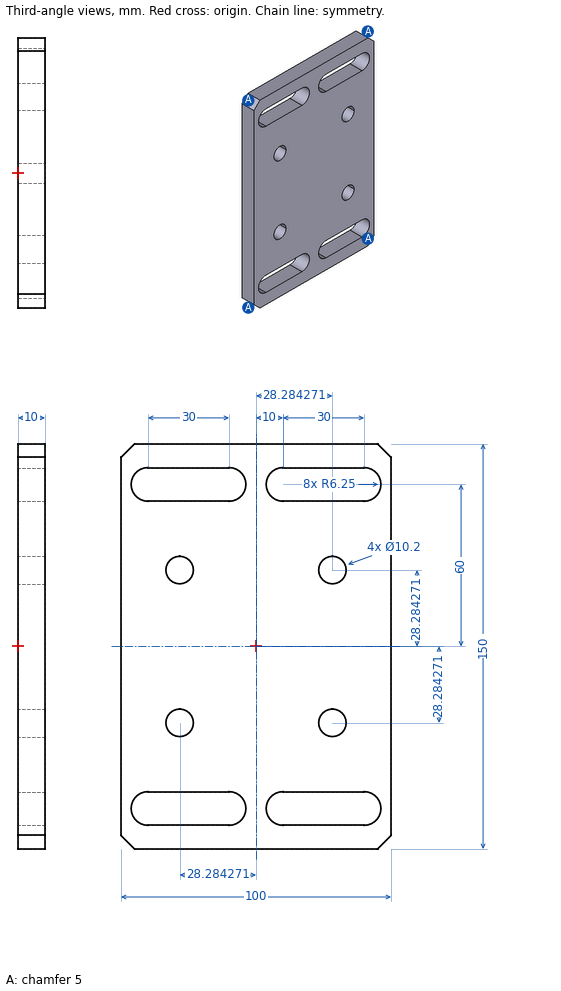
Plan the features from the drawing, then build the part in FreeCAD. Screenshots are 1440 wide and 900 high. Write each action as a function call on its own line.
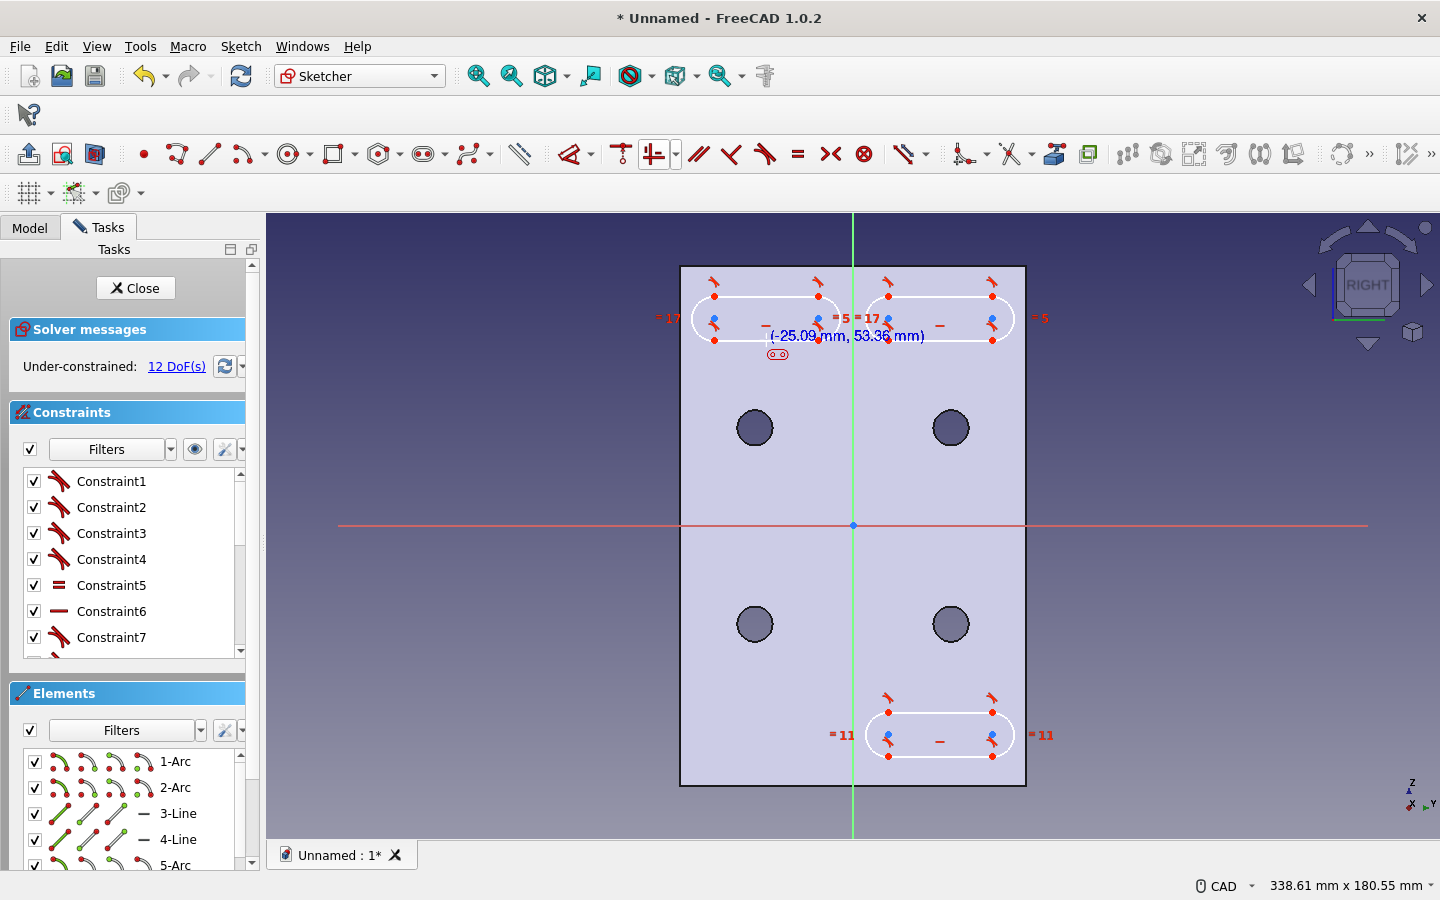
click(714, 734)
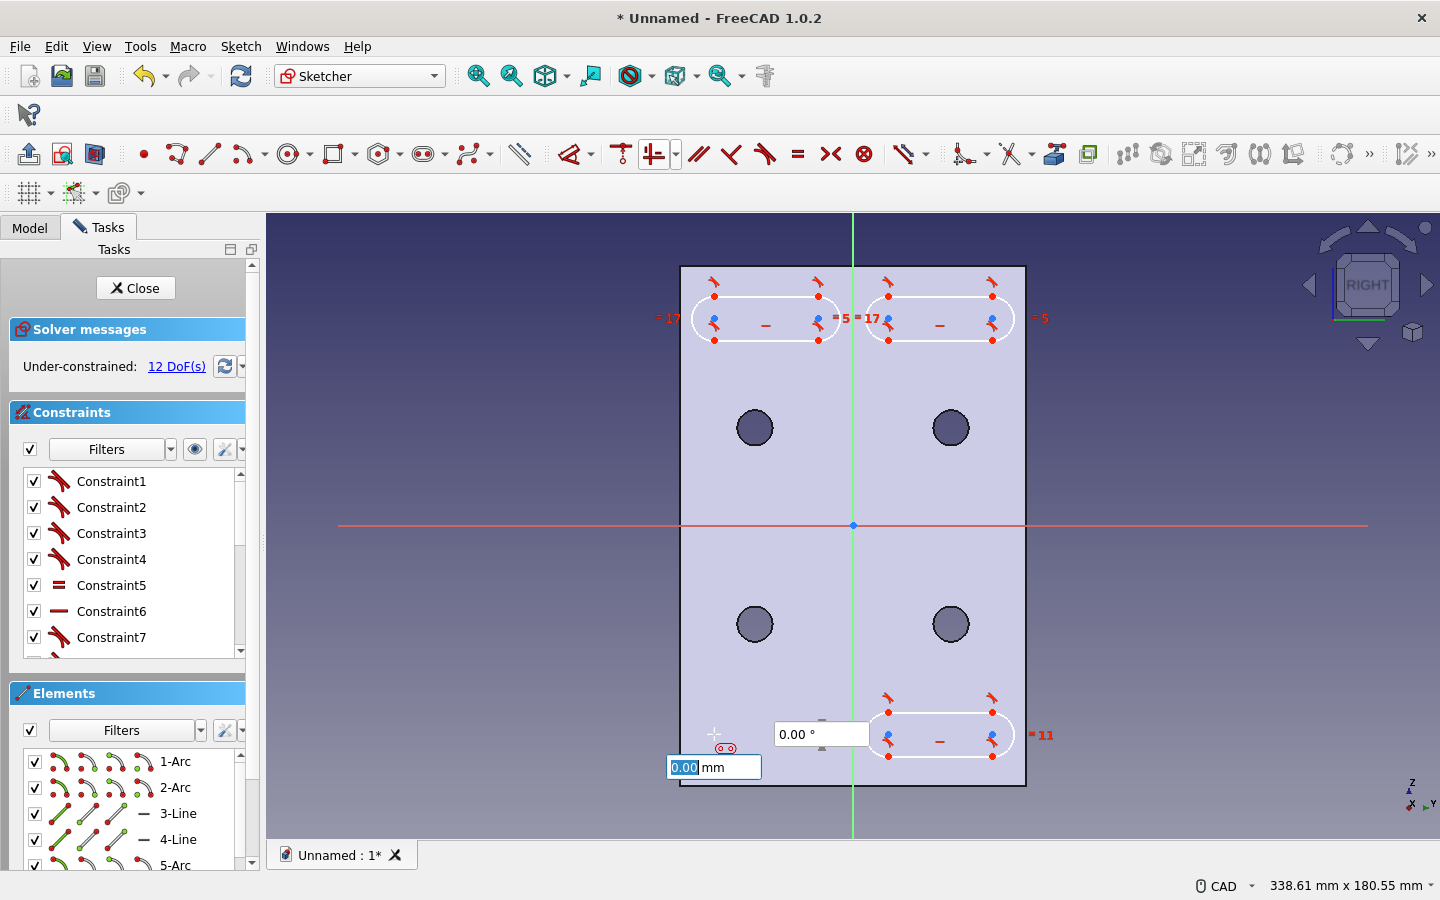
click(818, 734)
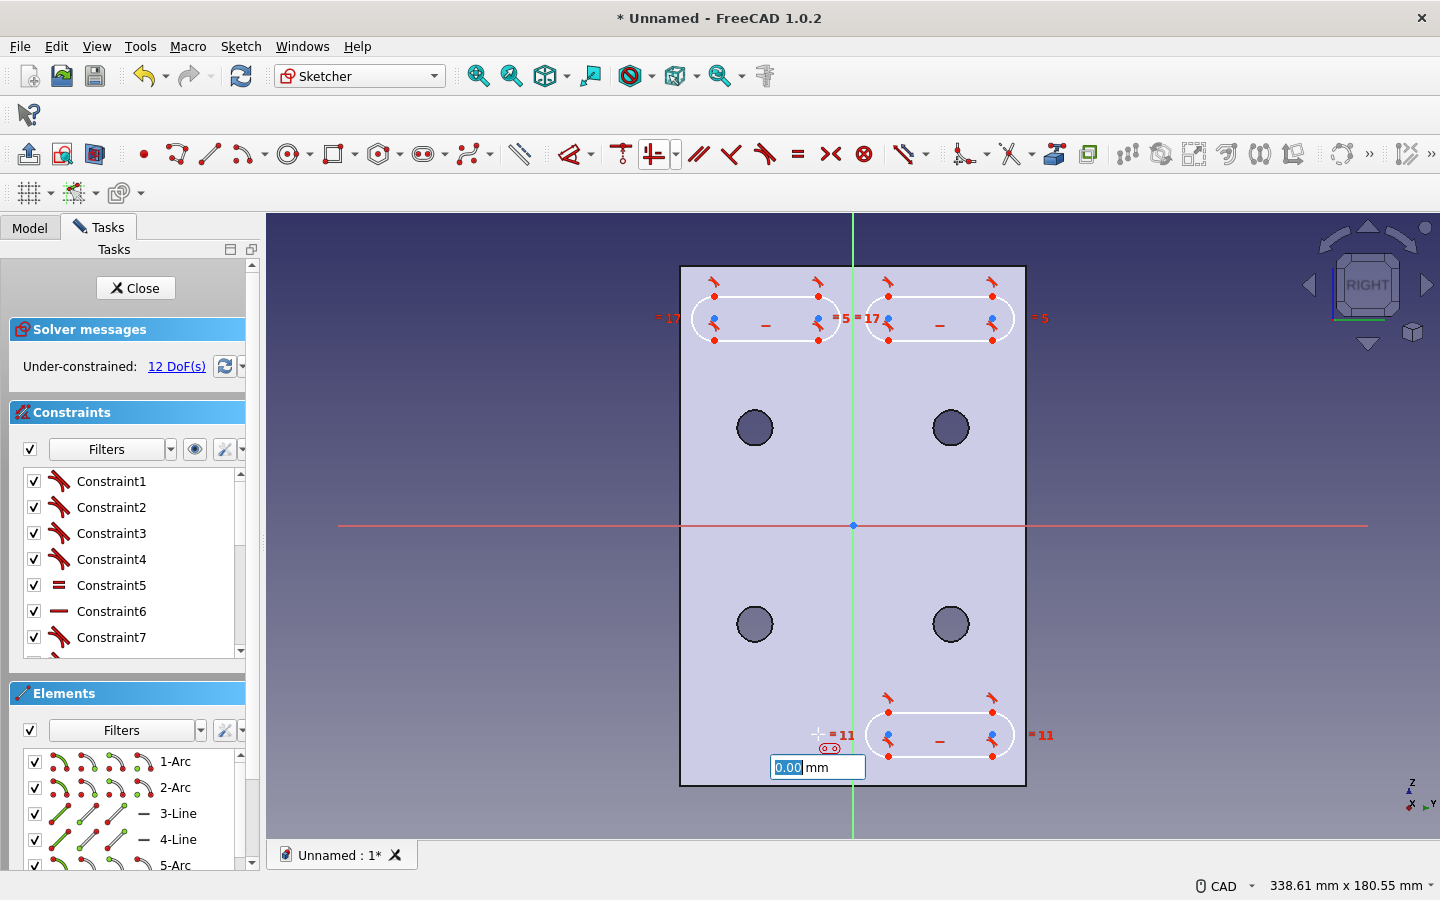
click(766, 712)
key(Escape)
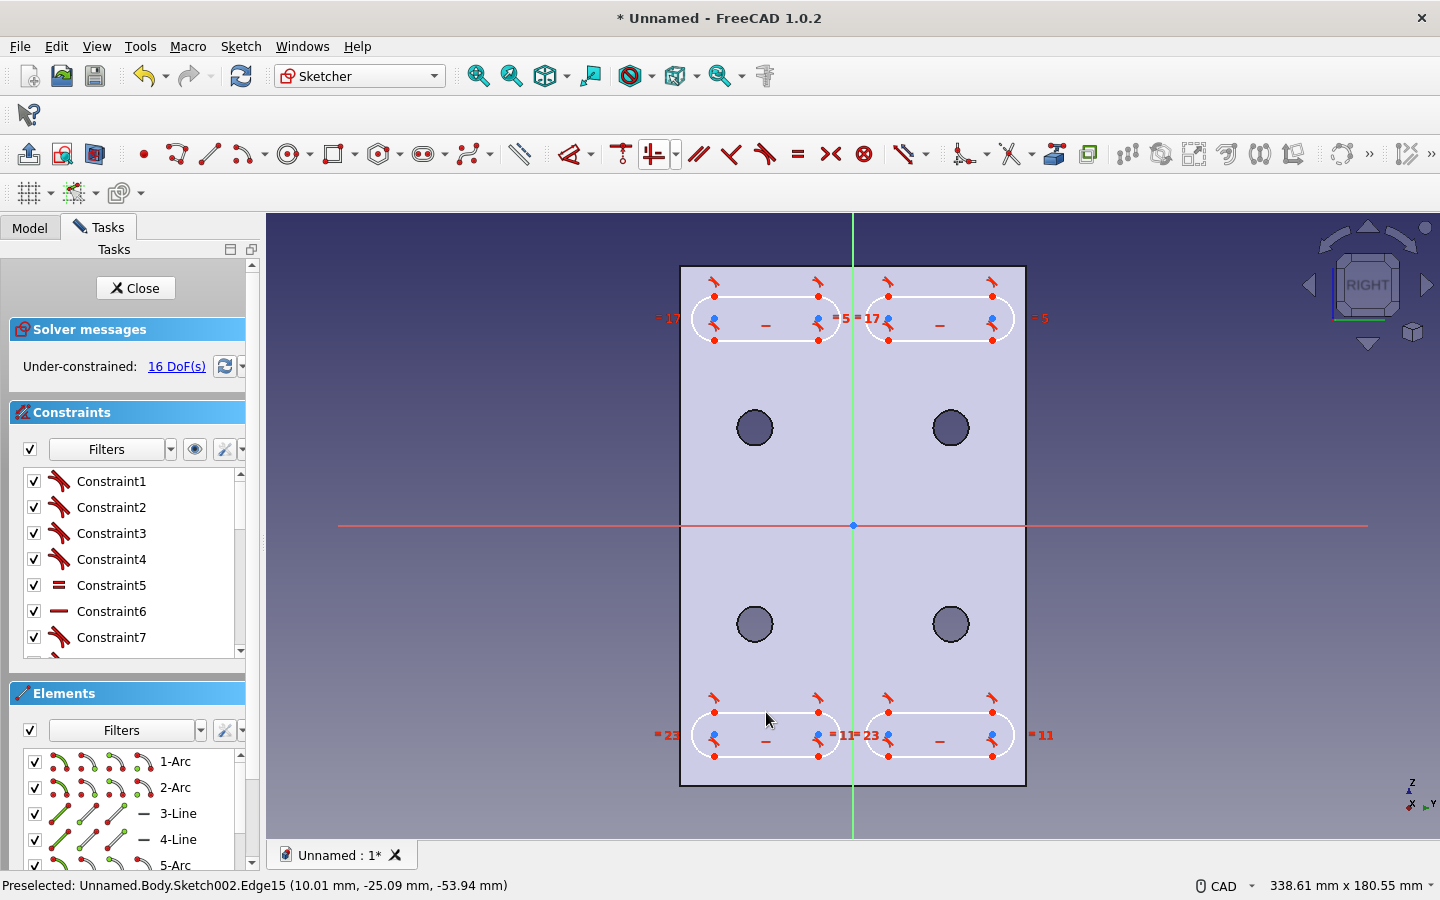
click(870, 306)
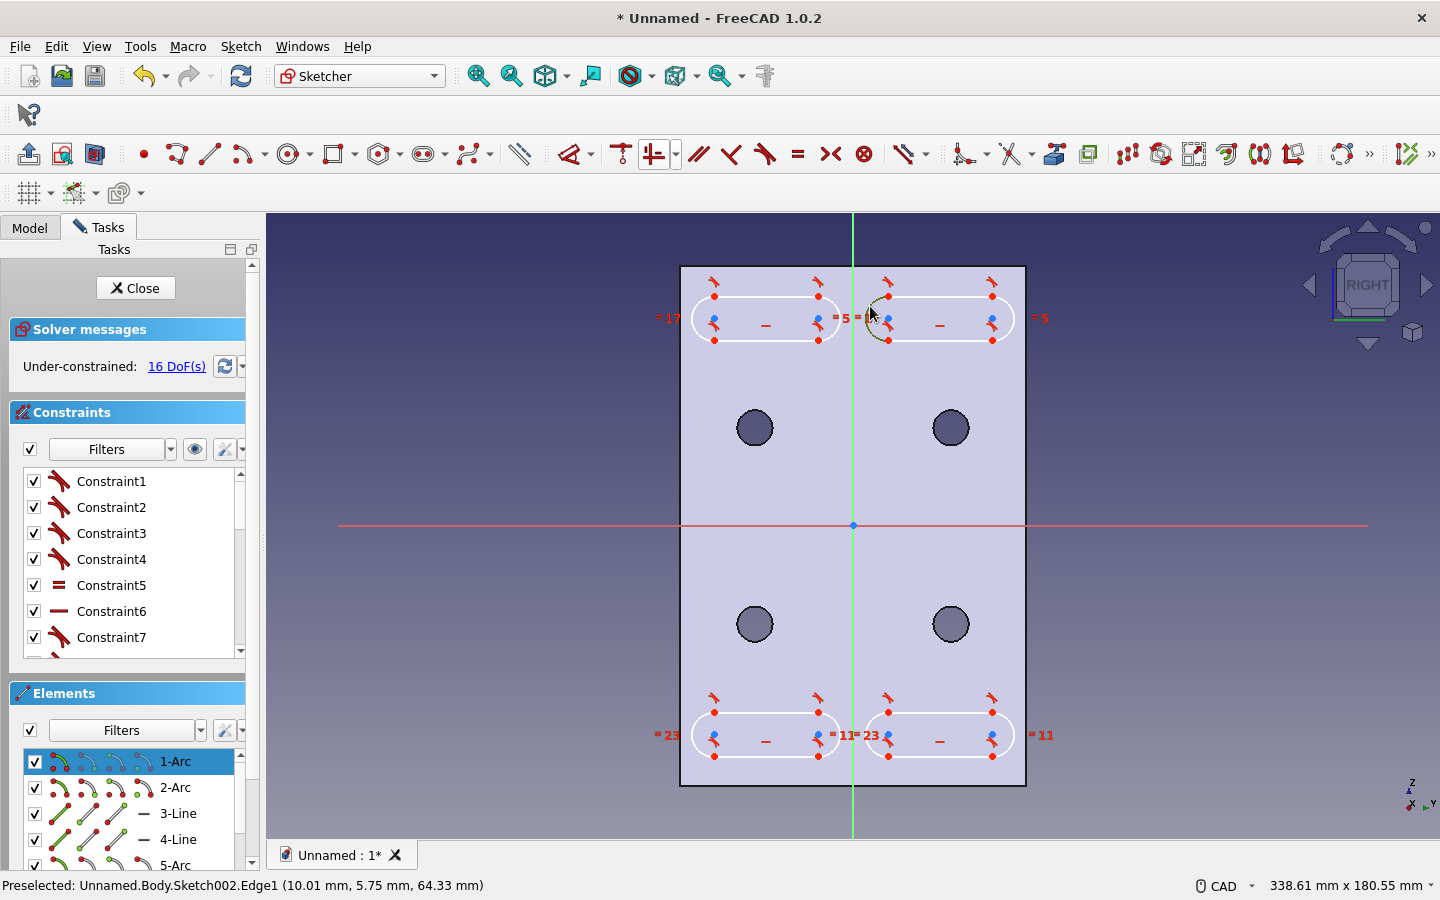
click(870, 722)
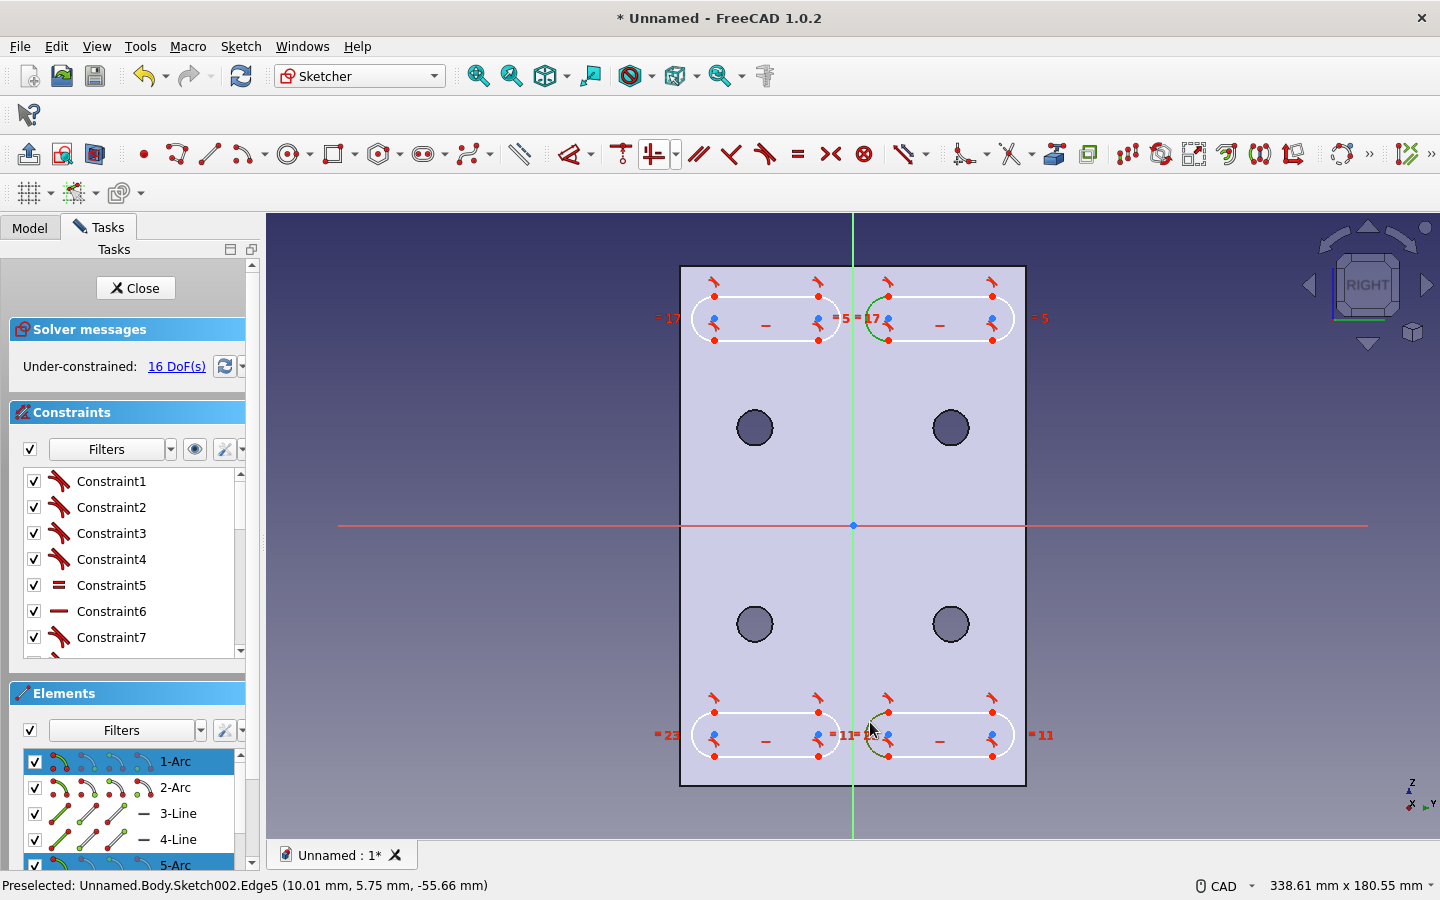
click(696, 306)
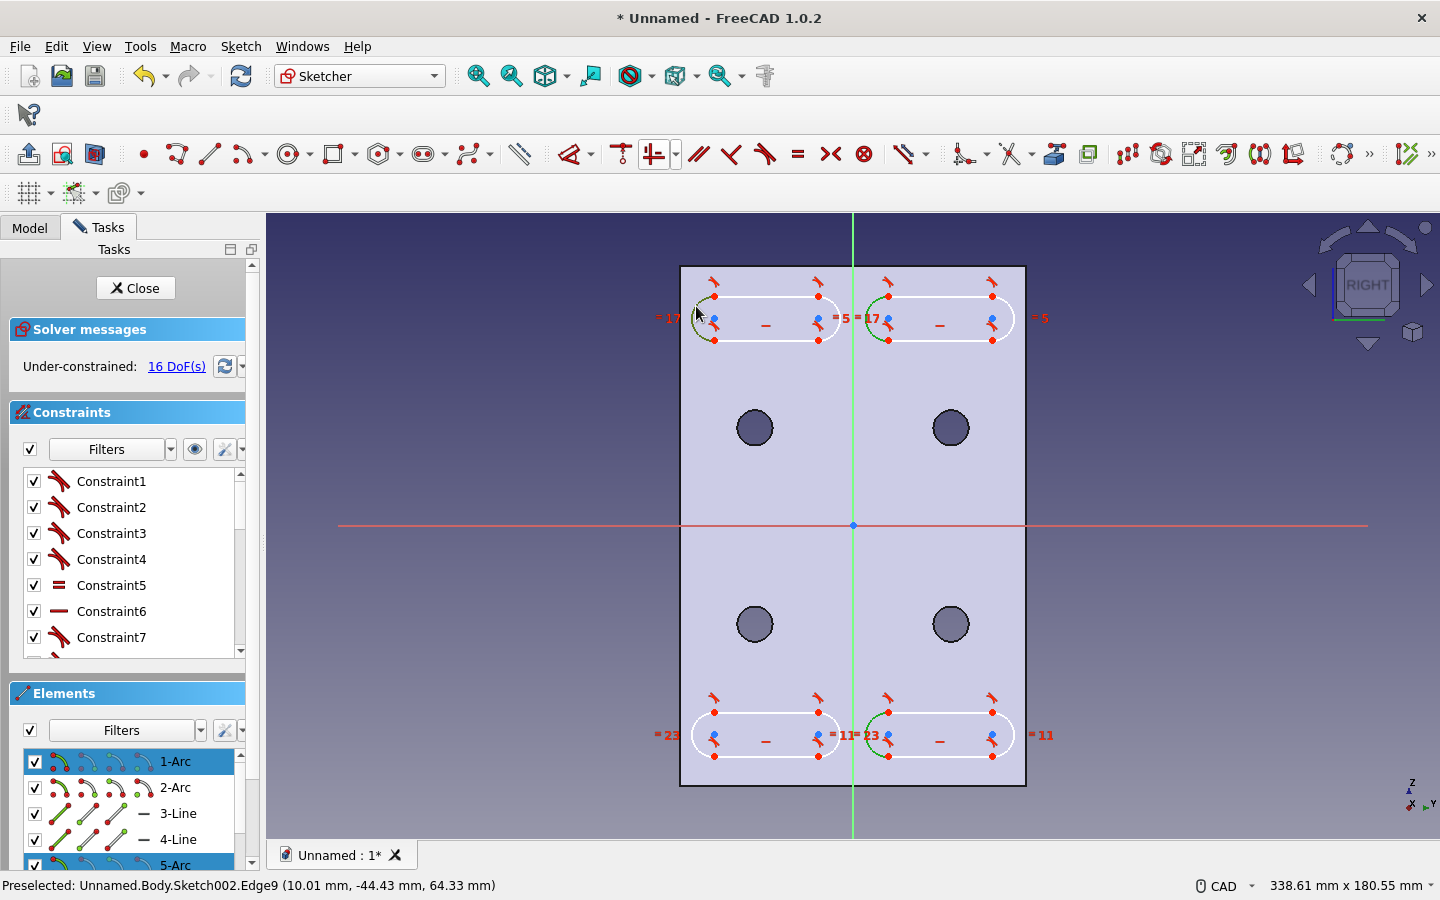
click(696, 722)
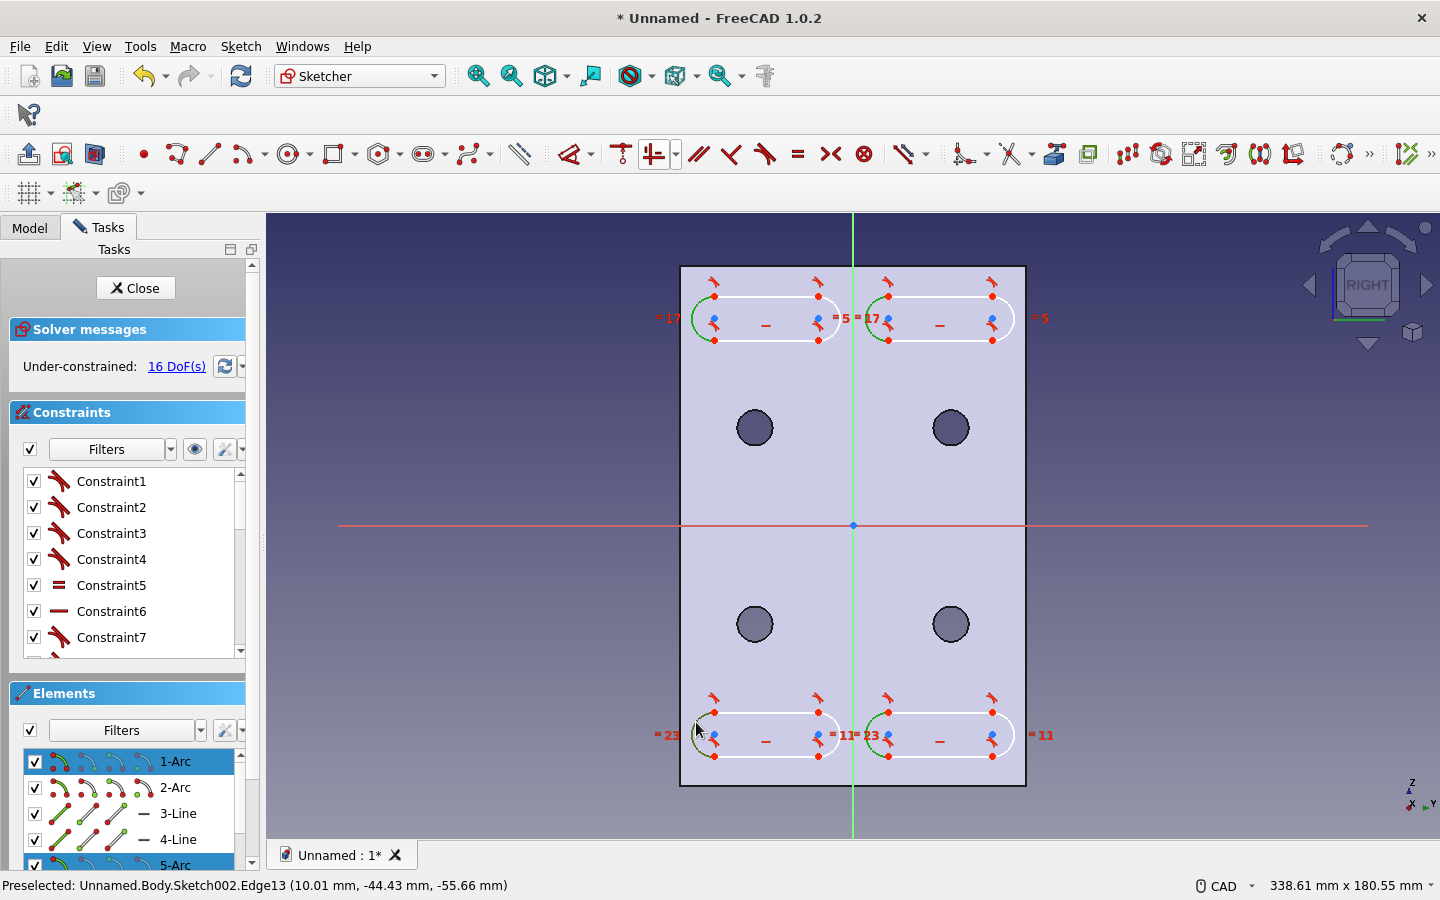
click(798, 154)